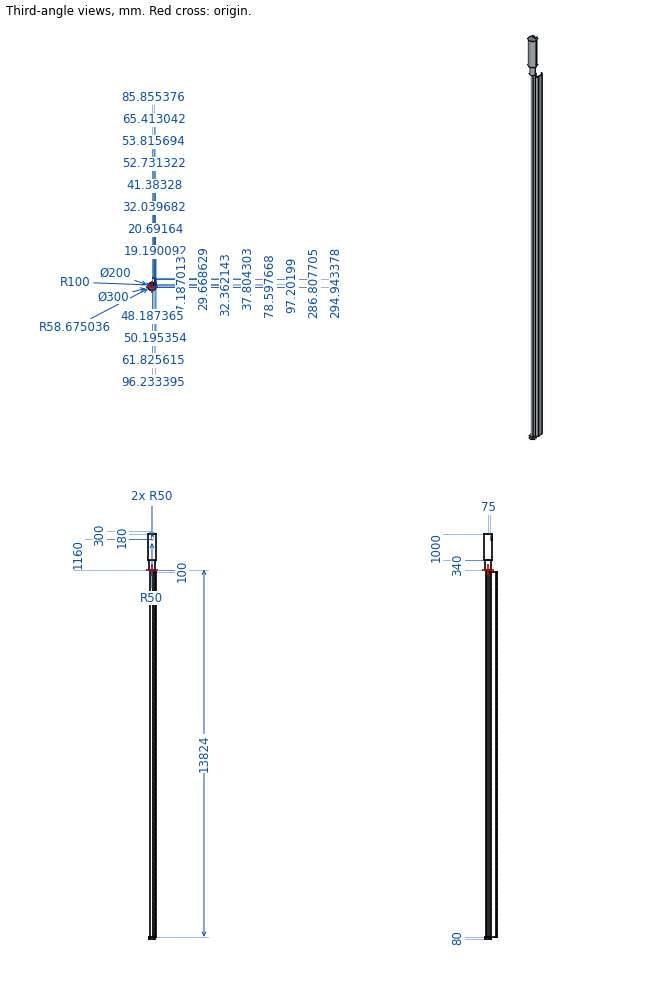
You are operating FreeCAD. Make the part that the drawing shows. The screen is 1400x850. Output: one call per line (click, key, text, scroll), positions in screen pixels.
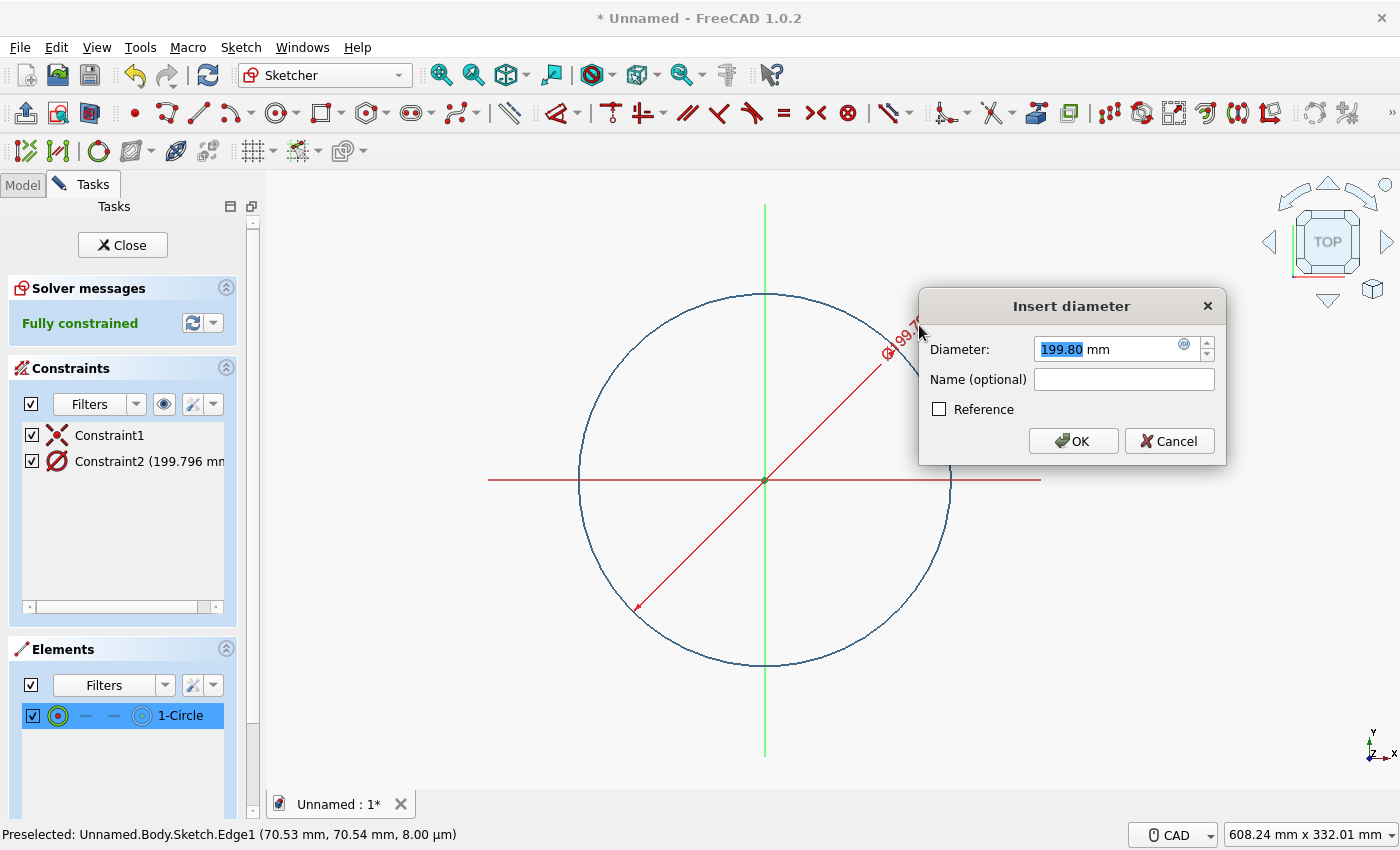
text(200)
key(Return)
key(Escape)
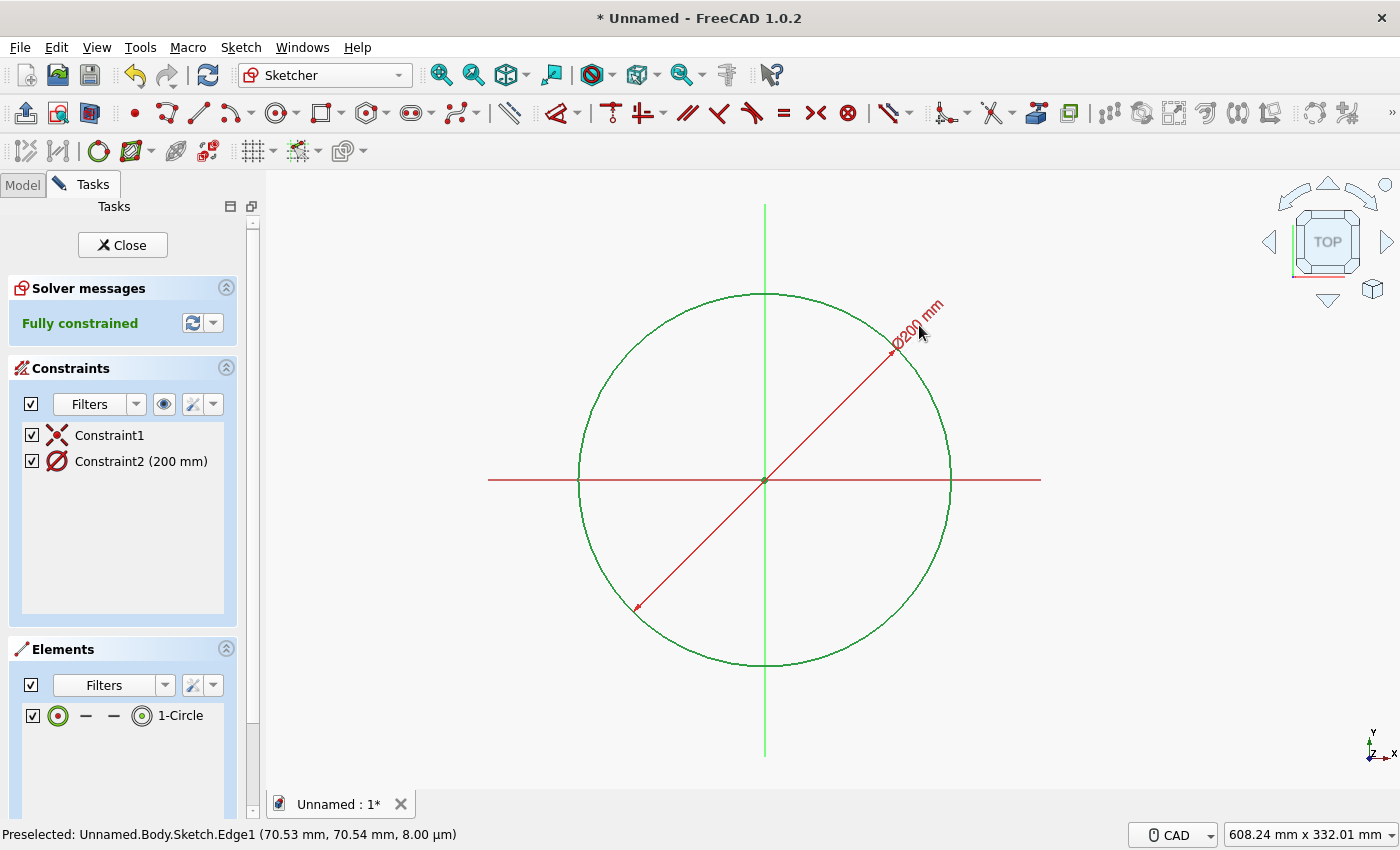
click(123, 245)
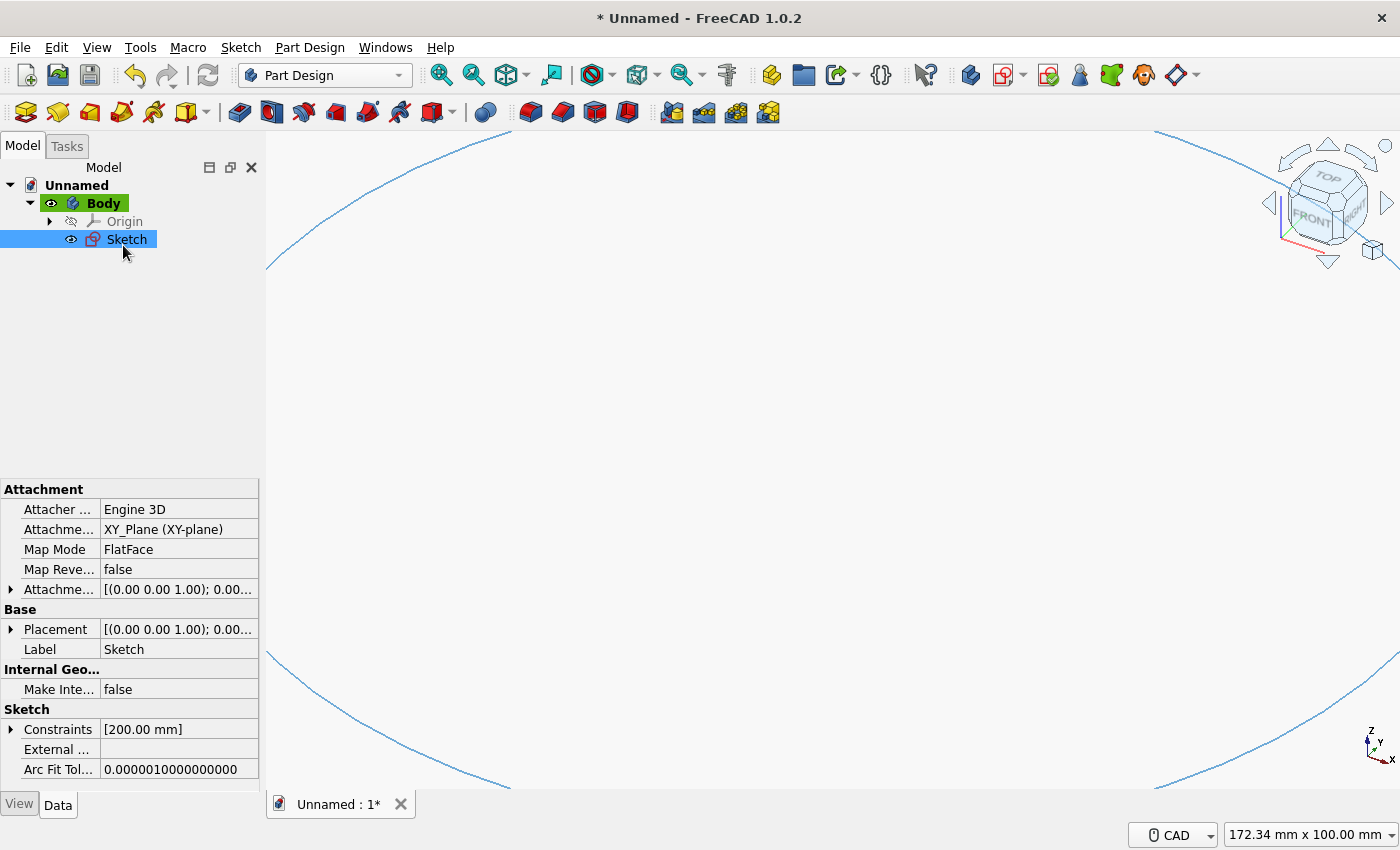
click(26, 112)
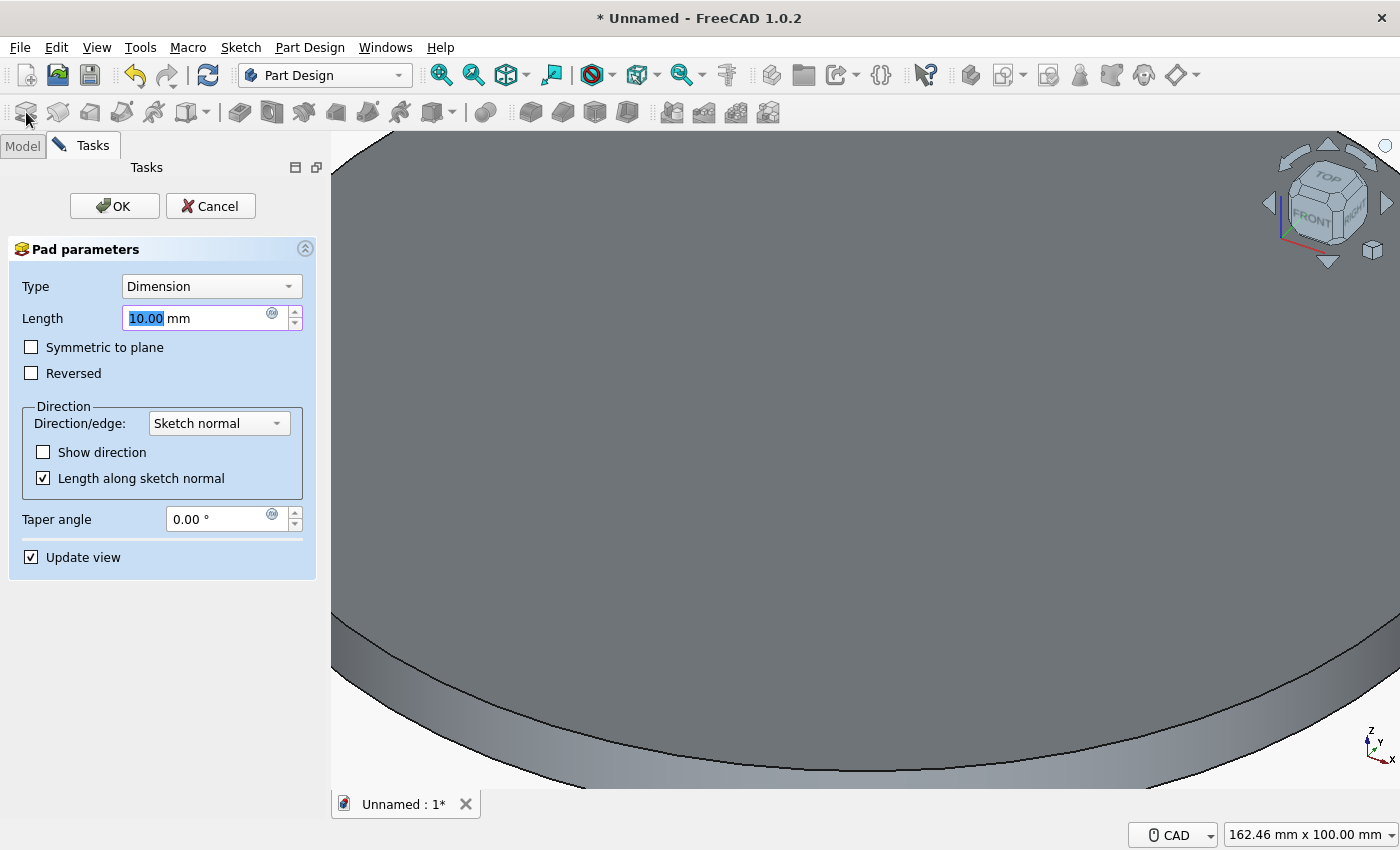
text(340)
key(Tab)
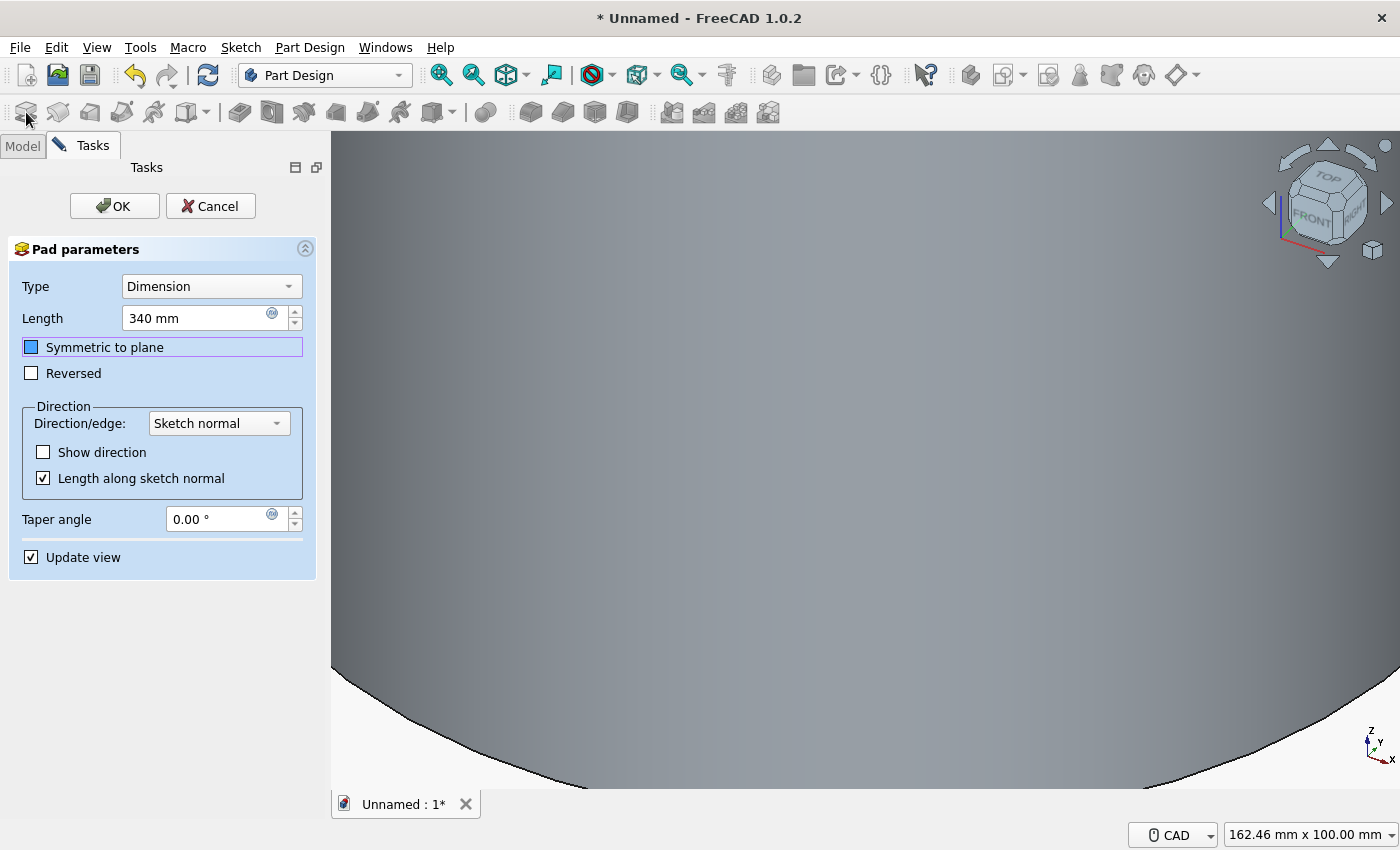
click(115, 206)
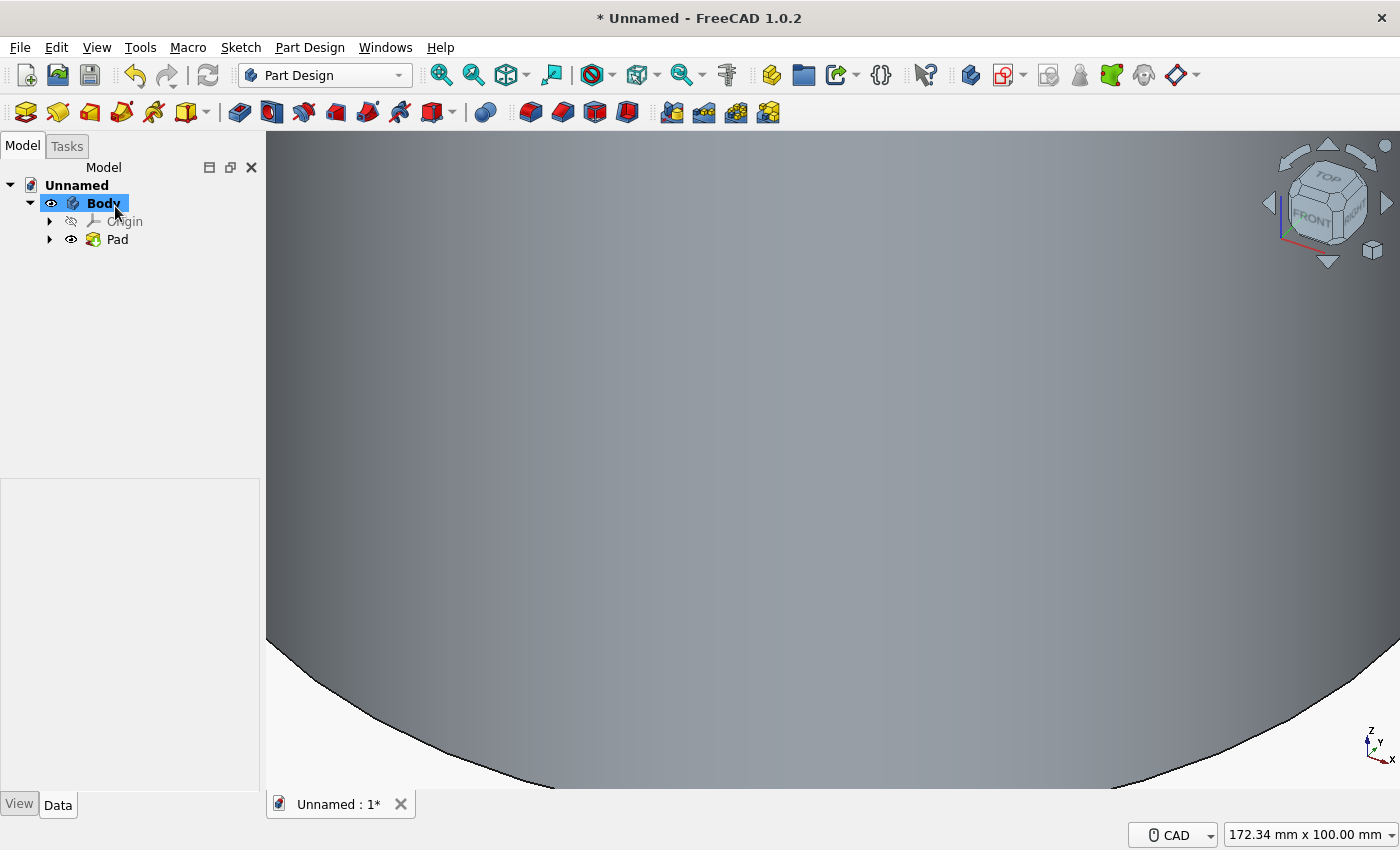
key(v)
key(f)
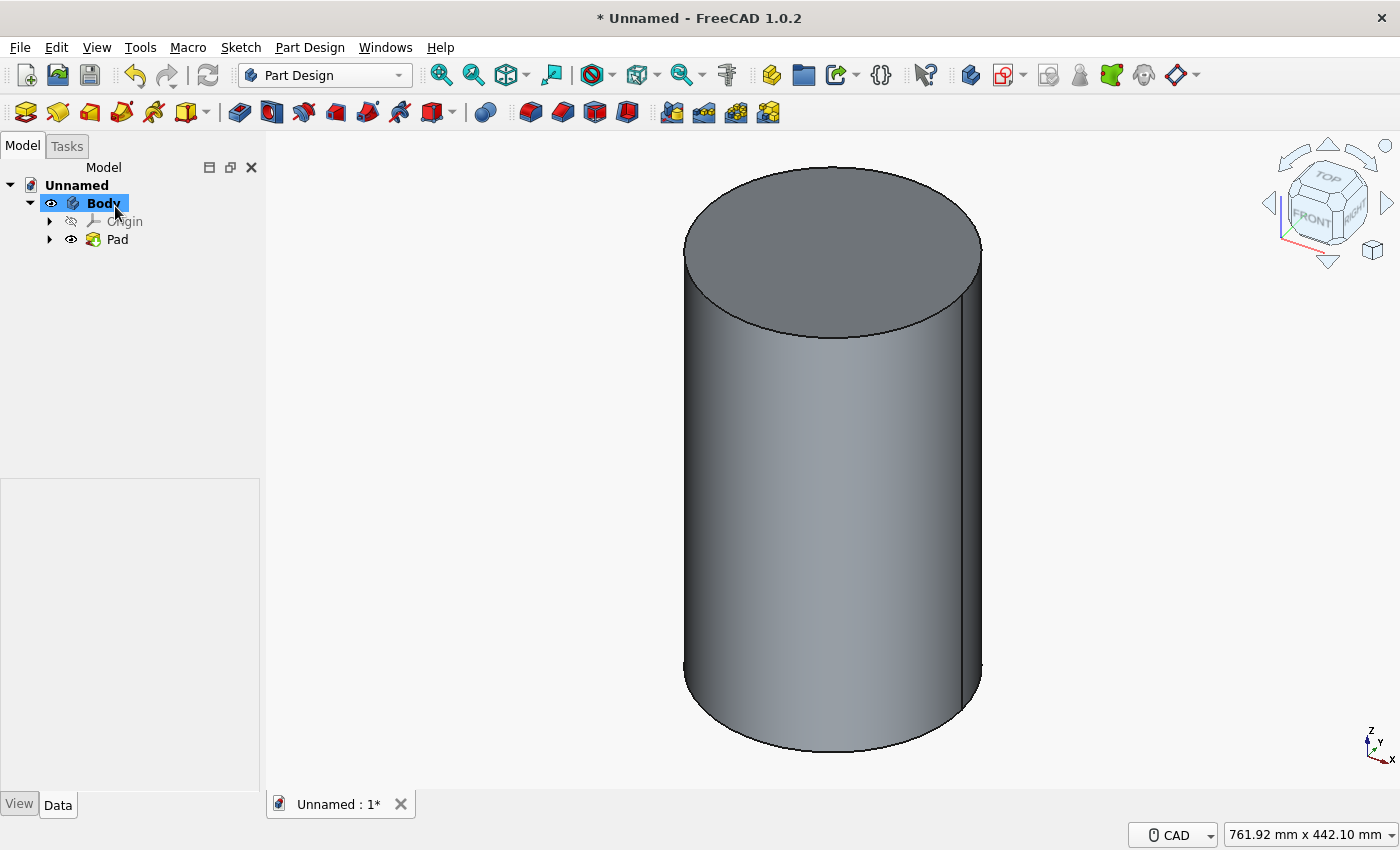
click(1004, 76)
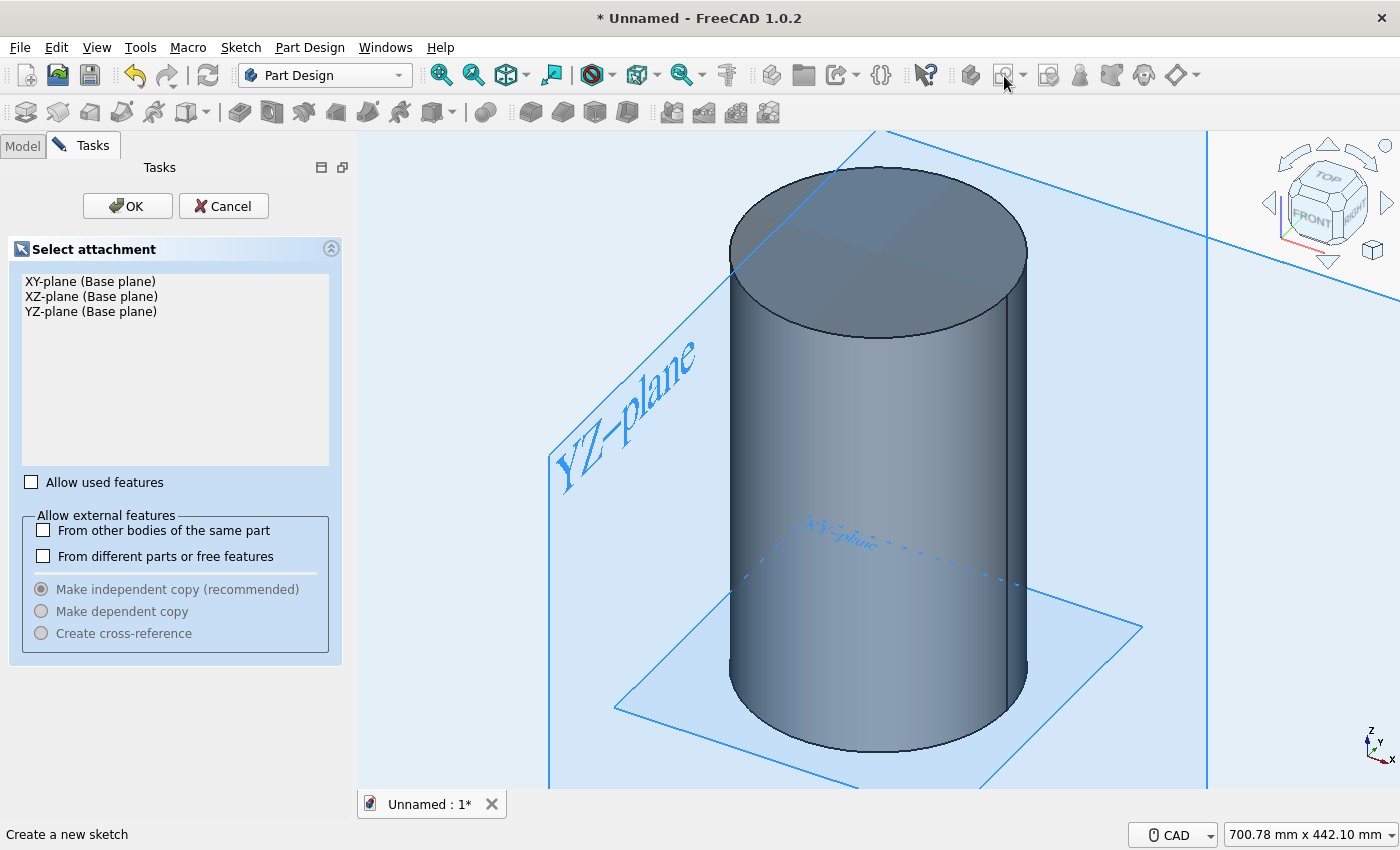
click(82, 282)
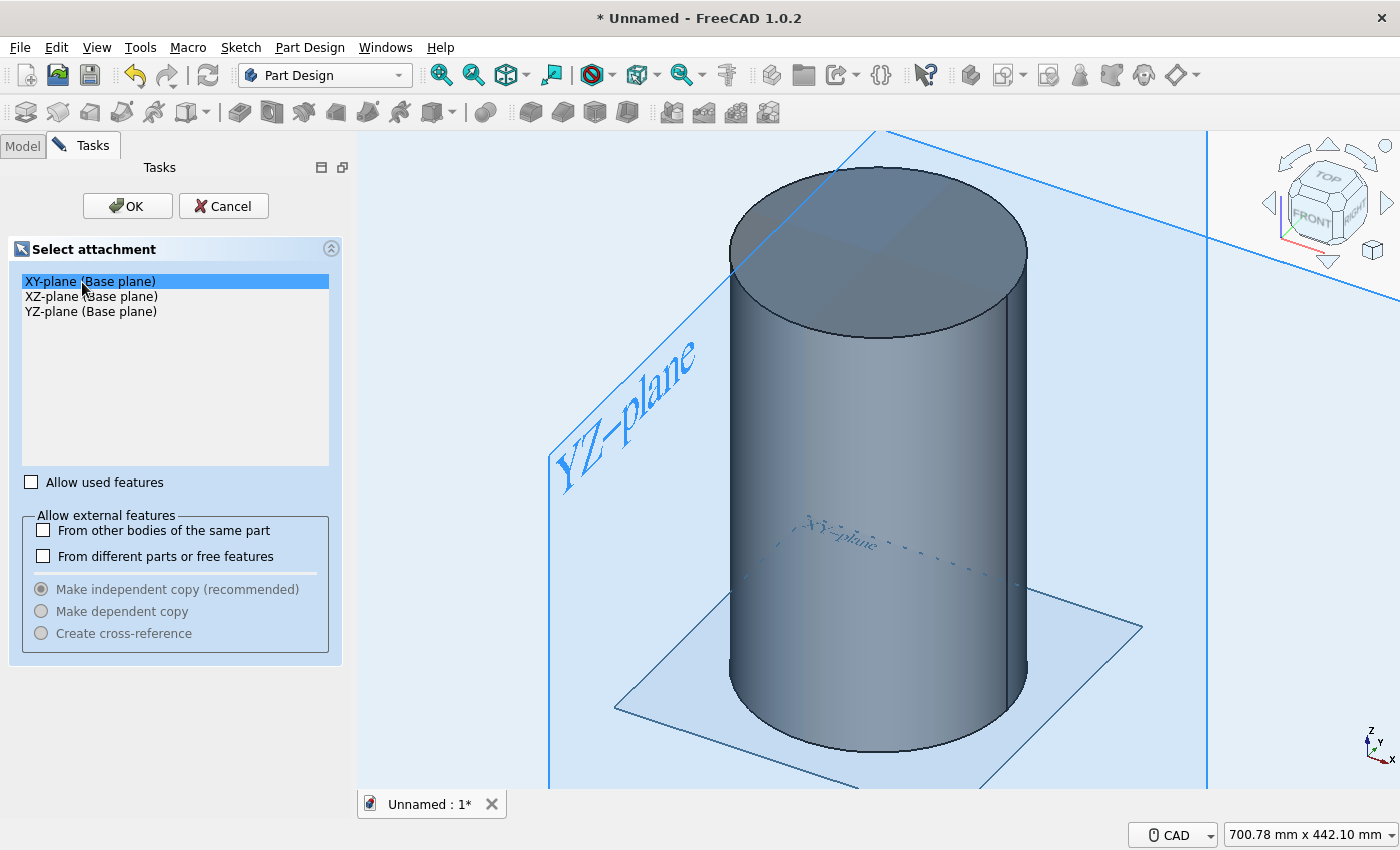
click(128, 206)